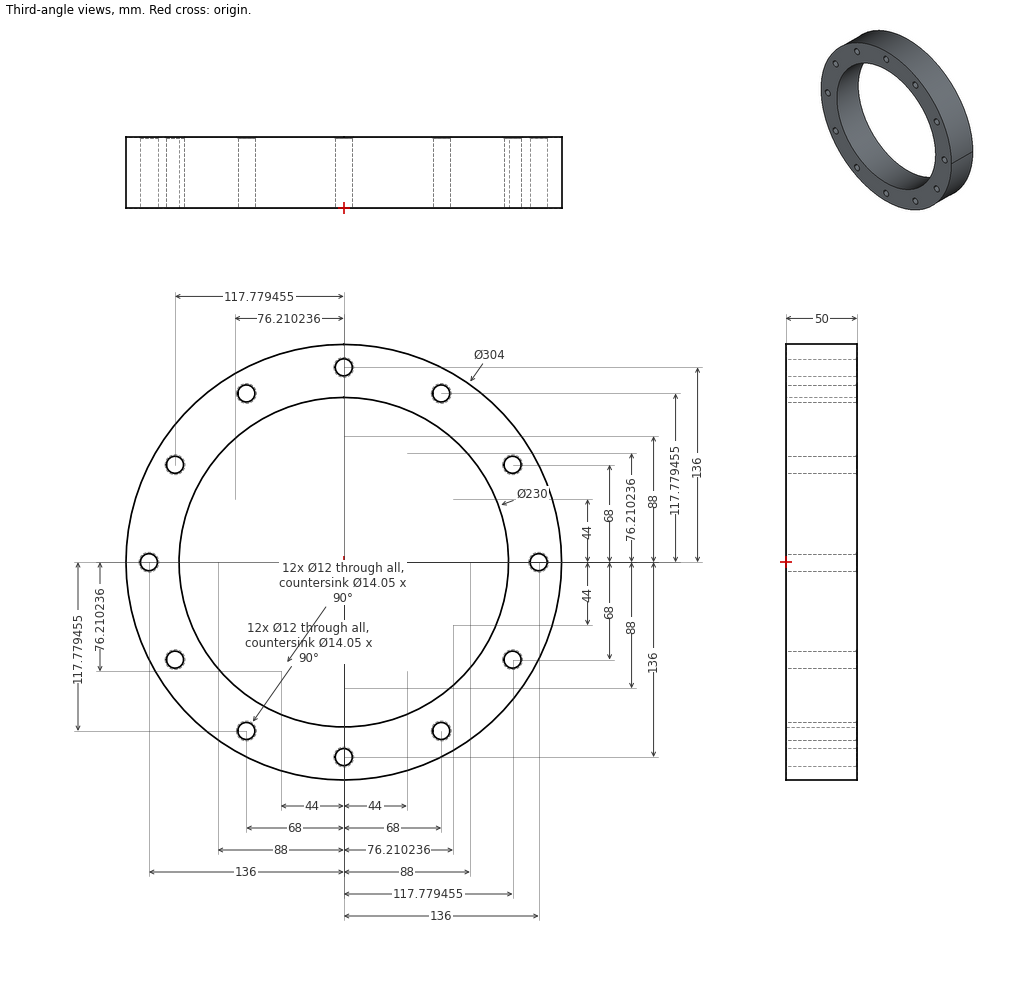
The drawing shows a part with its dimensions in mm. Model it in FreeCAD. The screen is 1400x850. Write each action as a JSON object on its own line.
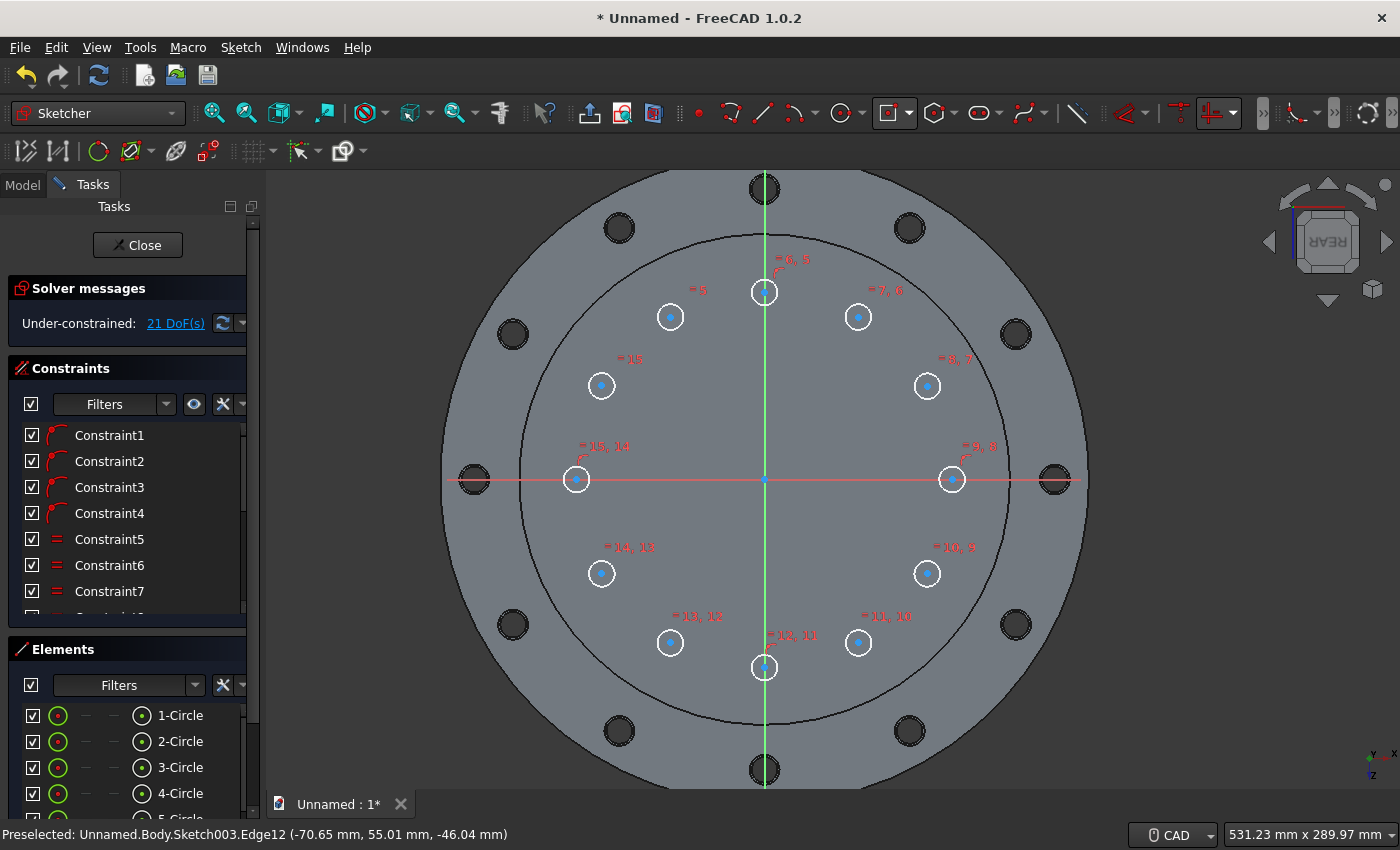
{"action": "left_click", "coordinate": [671, 317]}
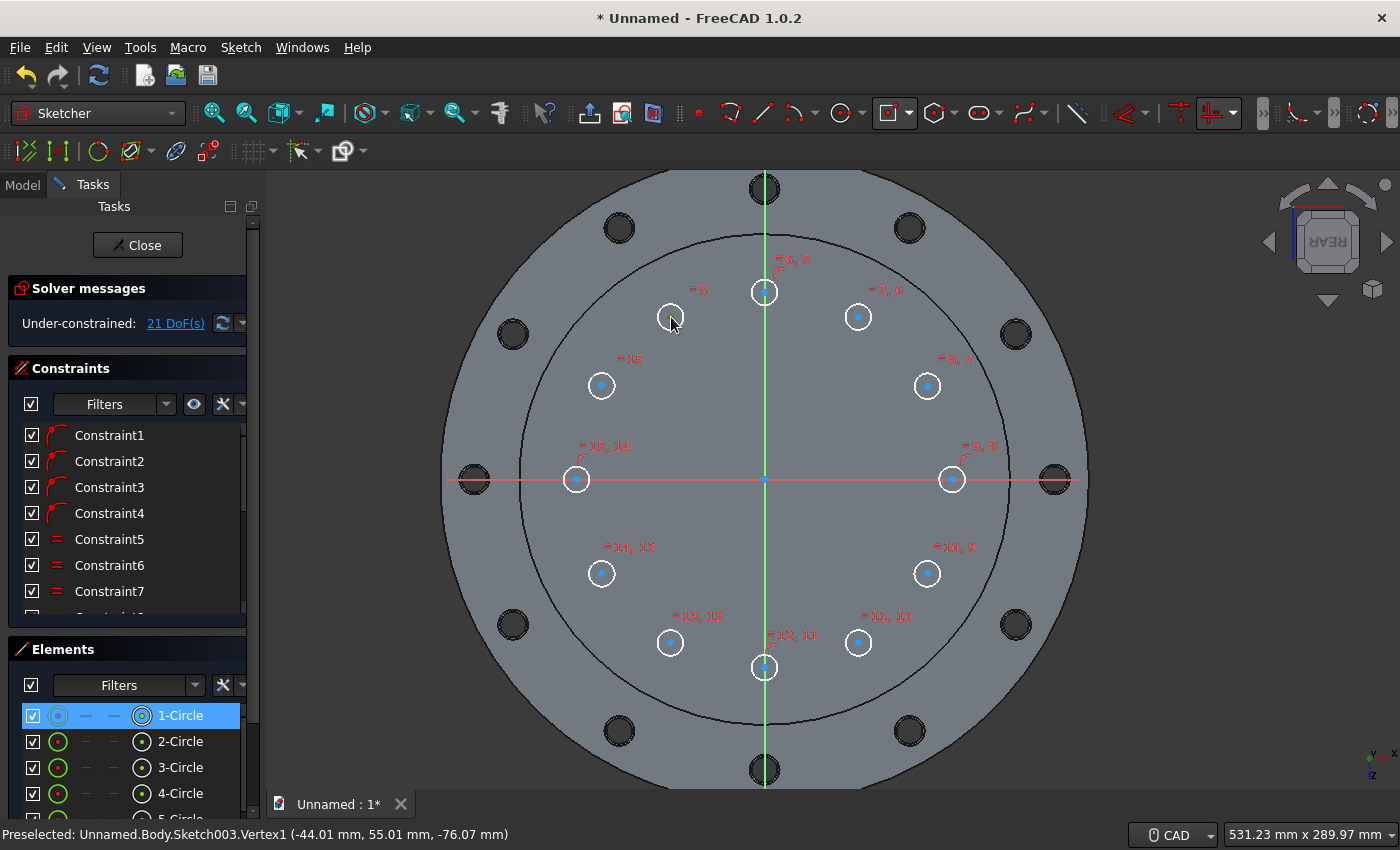
{"action": "left_click", "coordinate": [858, 317]}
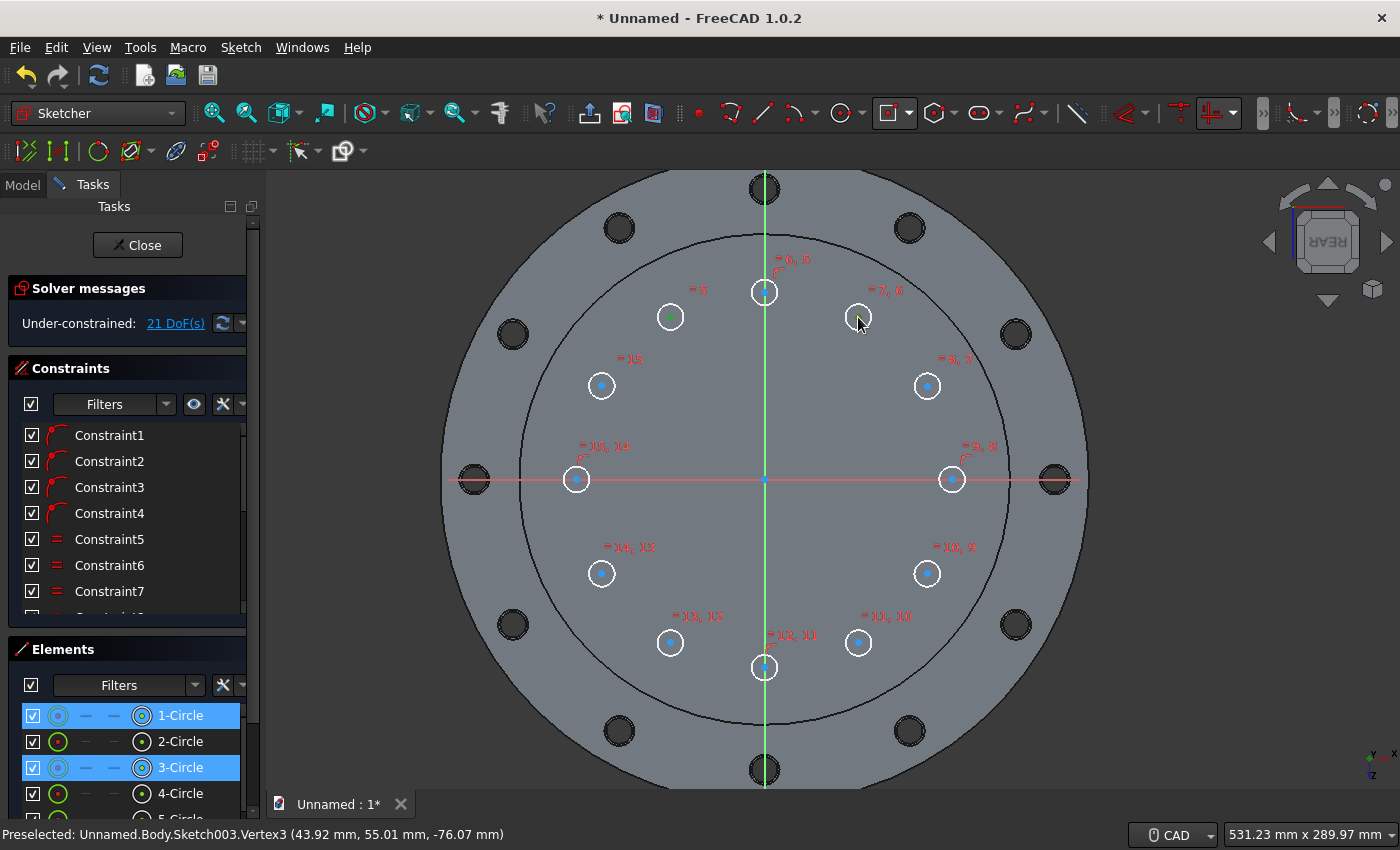
{"action": "left_click", "coordinate": [1236, 114]}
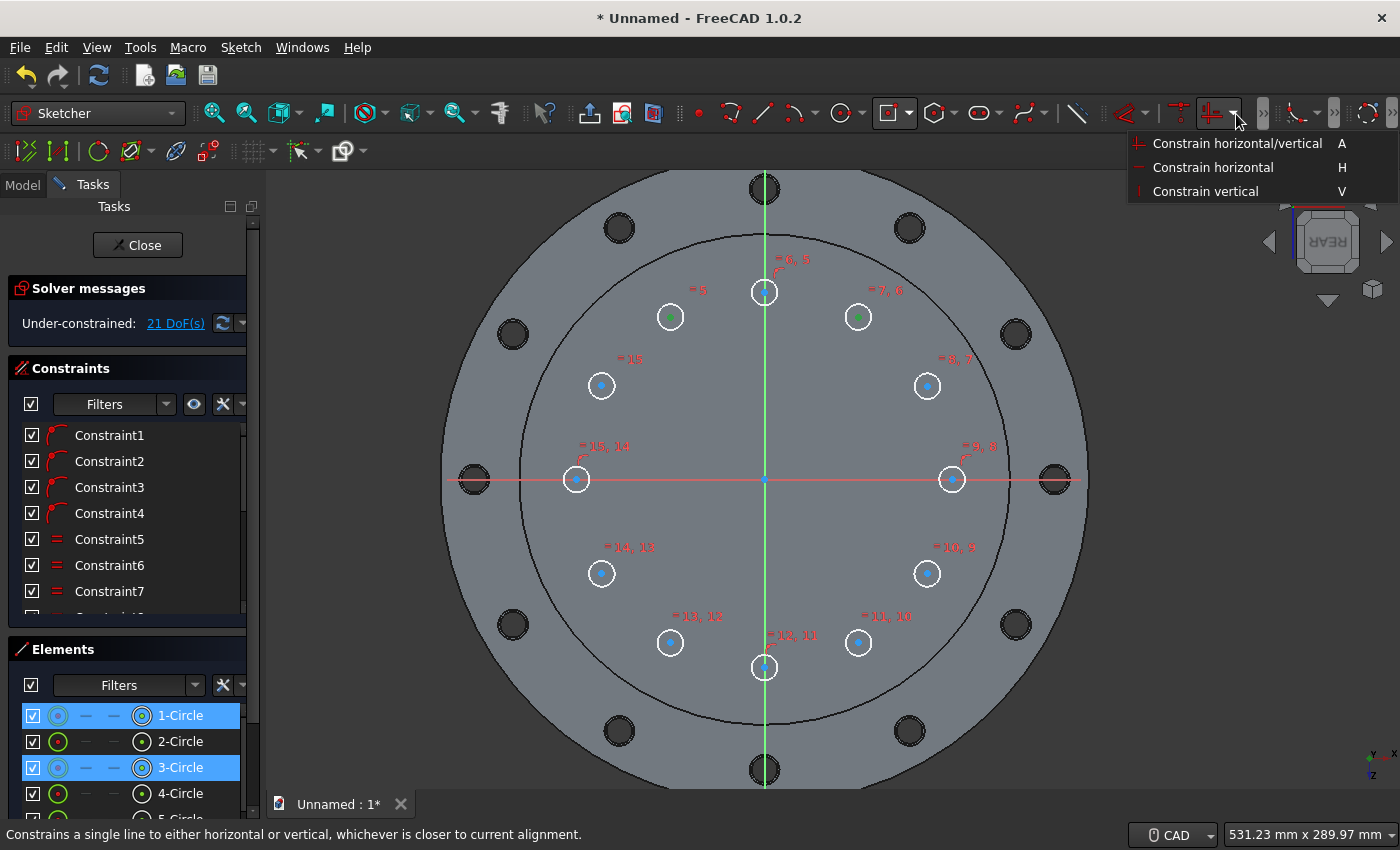
{"action": "left_click", "coordinate": [1263, 167]}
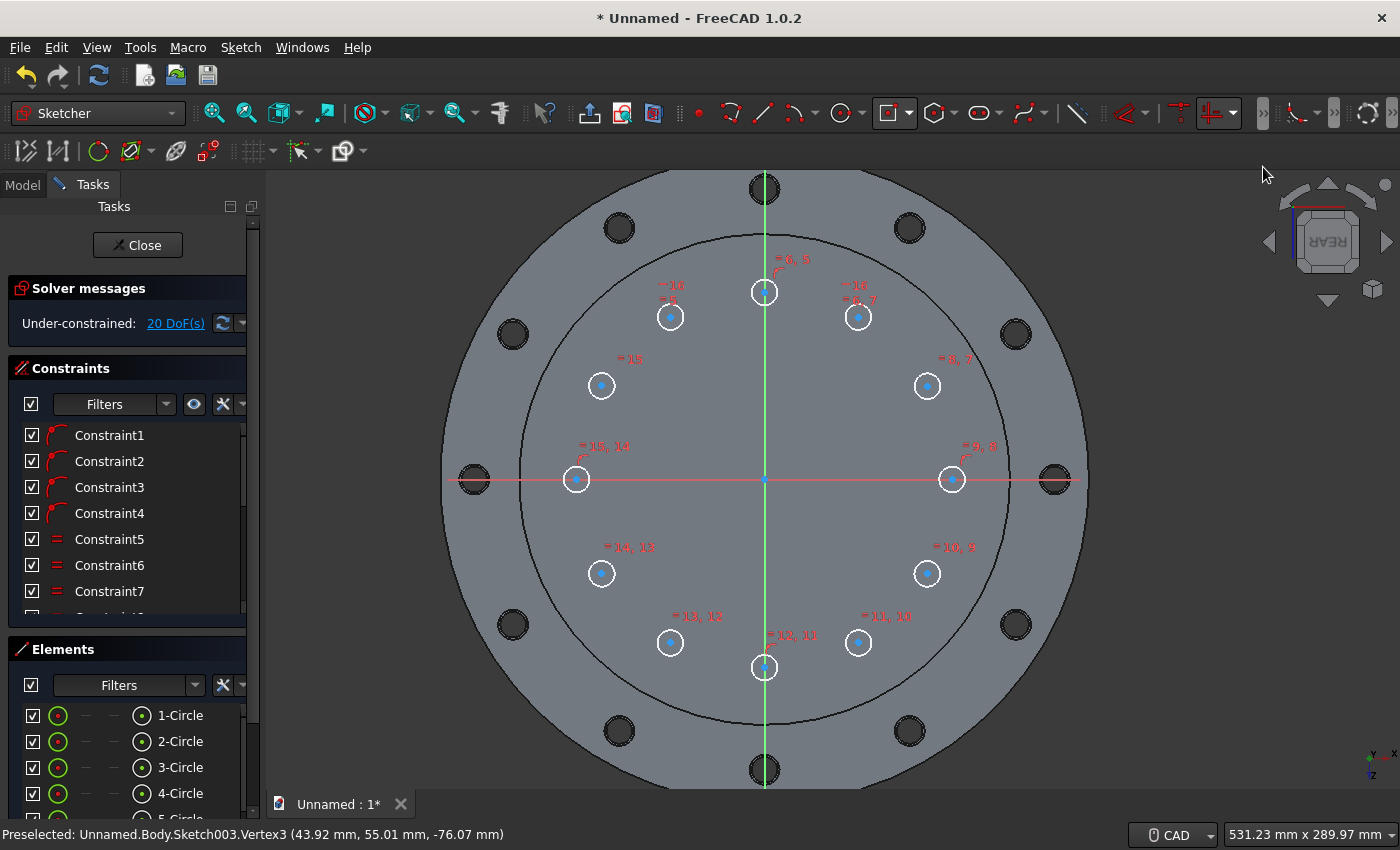
{"action": "left_click", "coordinate": [927, 386]}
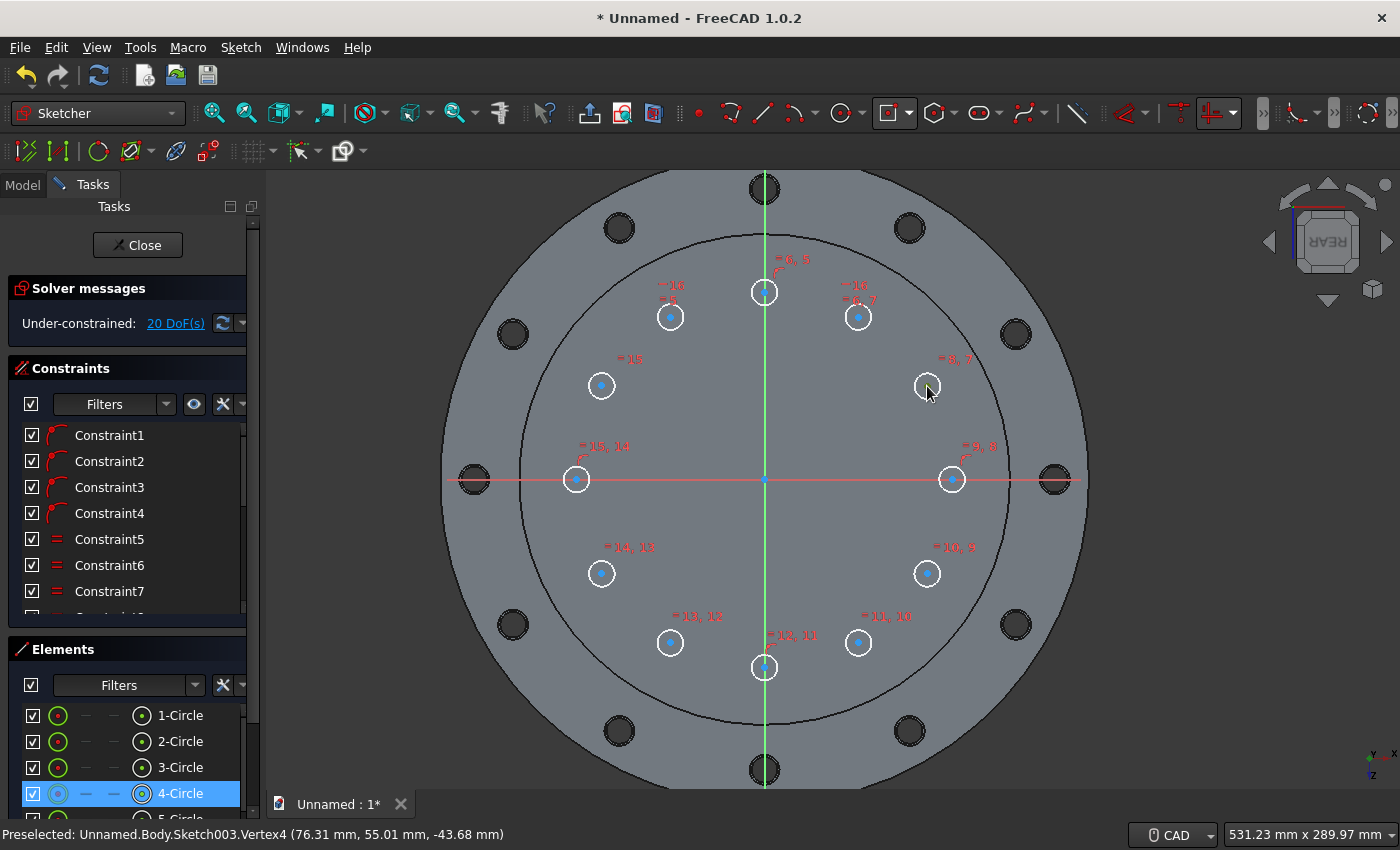
{"action": "left_click", "coordinate": [927, 574]}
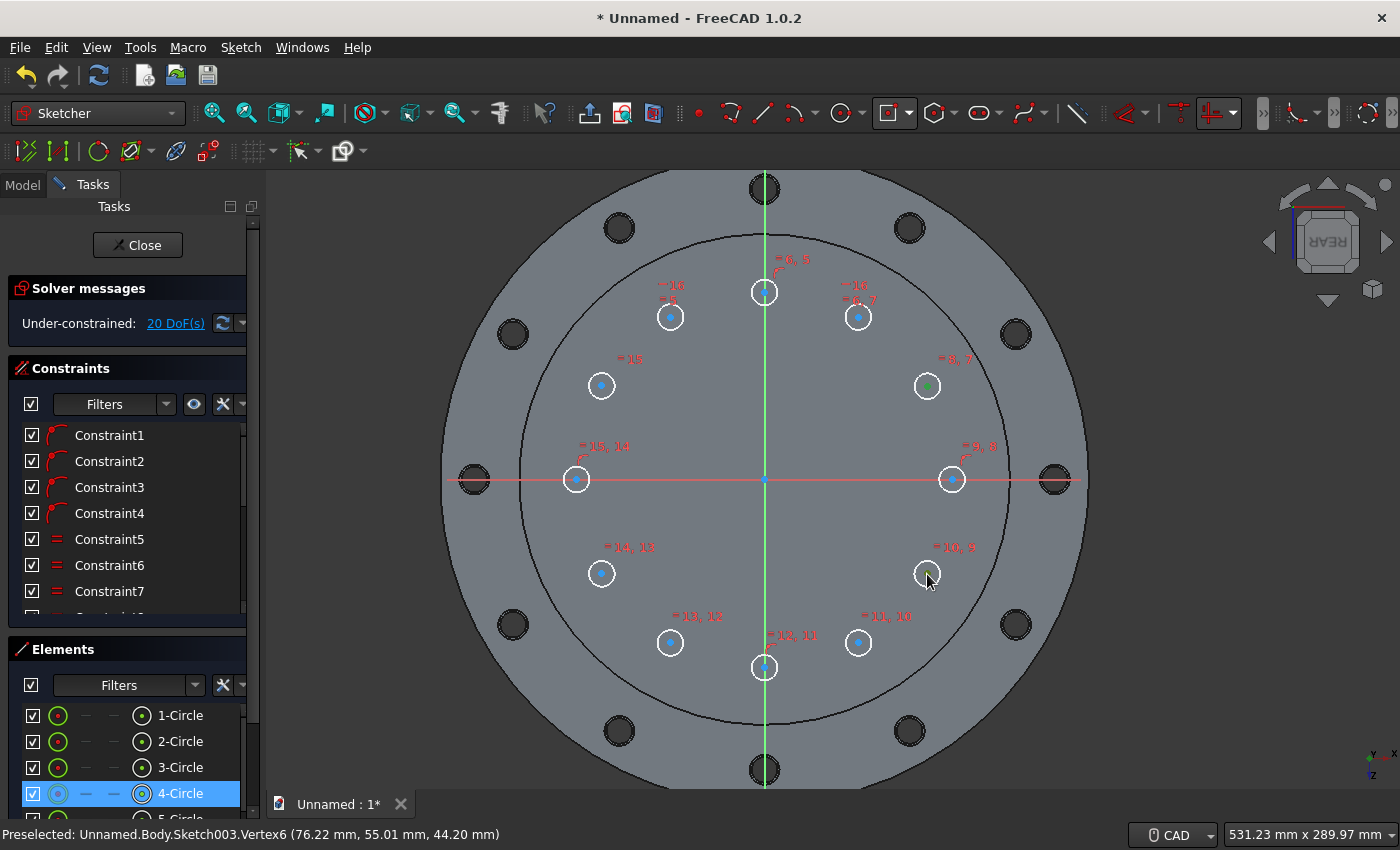
{"action": "key", "text": "v"}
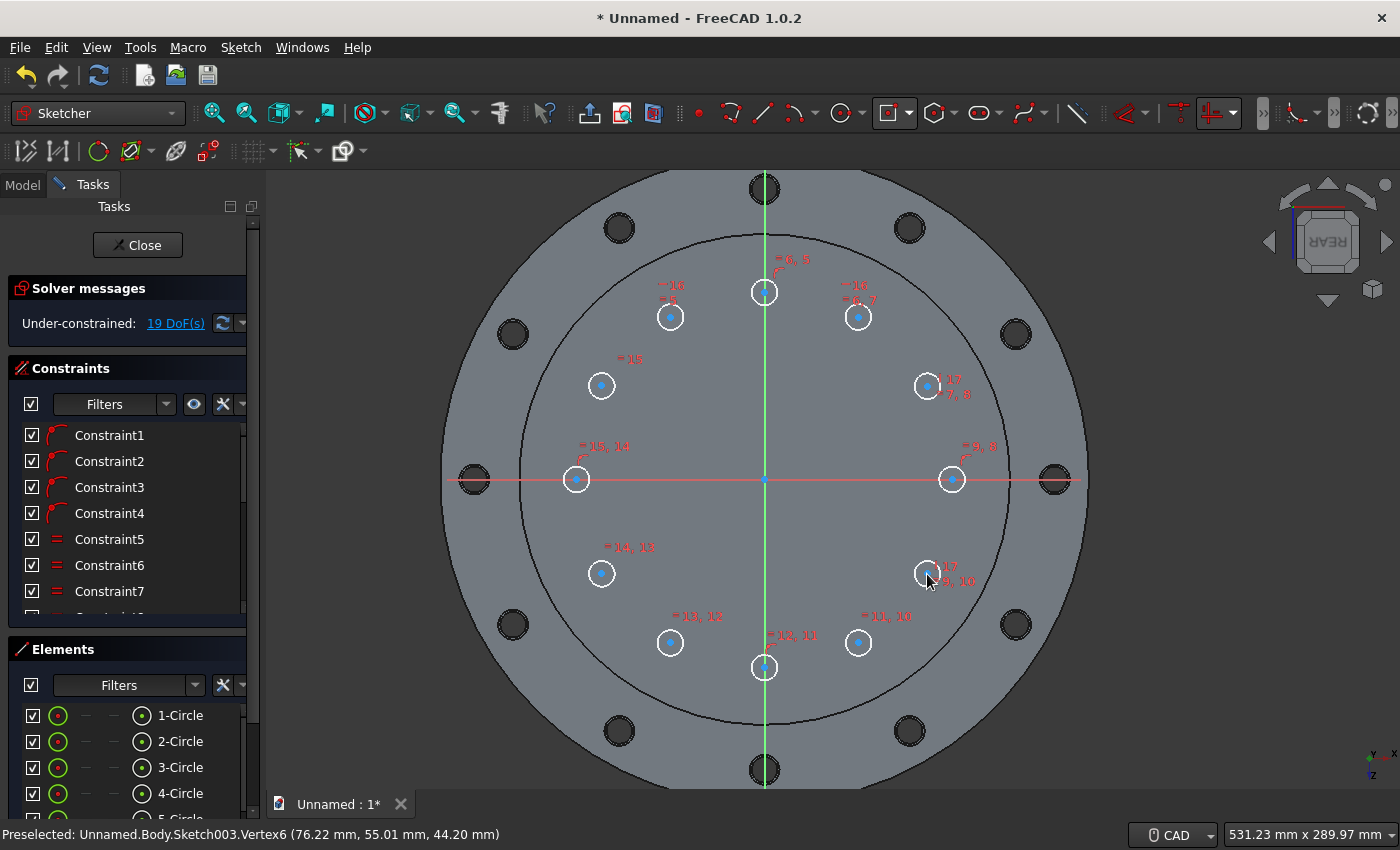
{"action": "left_click", "coordinate": [858, 317]}